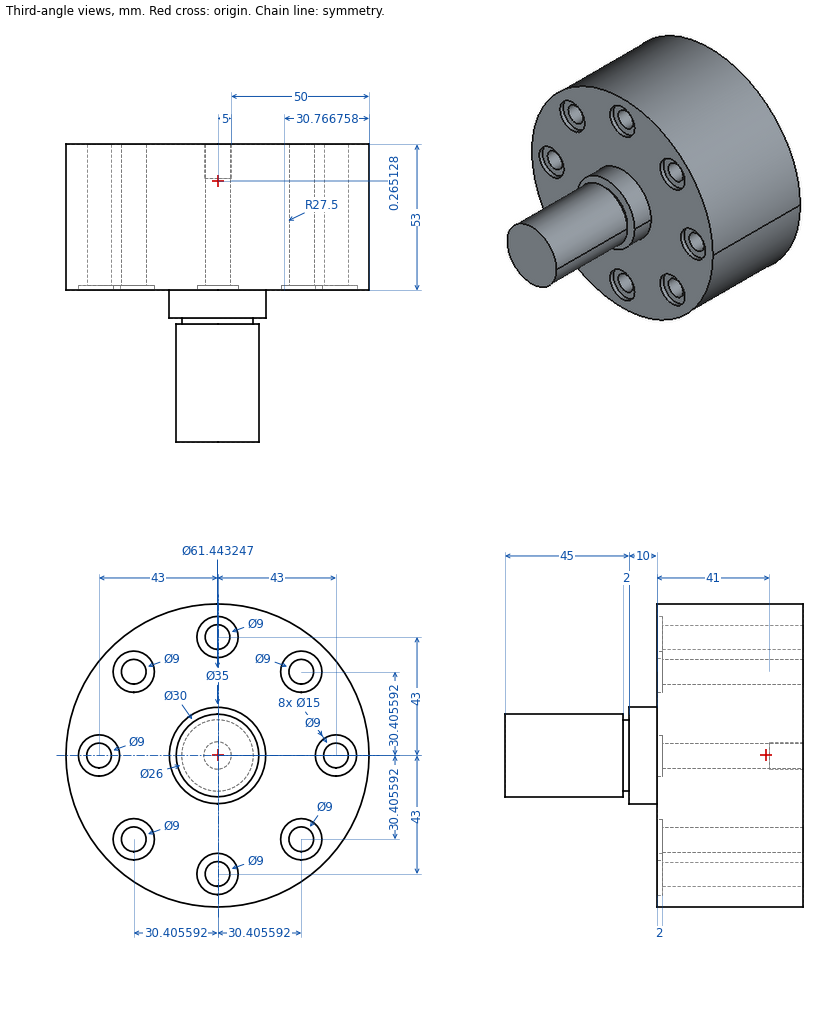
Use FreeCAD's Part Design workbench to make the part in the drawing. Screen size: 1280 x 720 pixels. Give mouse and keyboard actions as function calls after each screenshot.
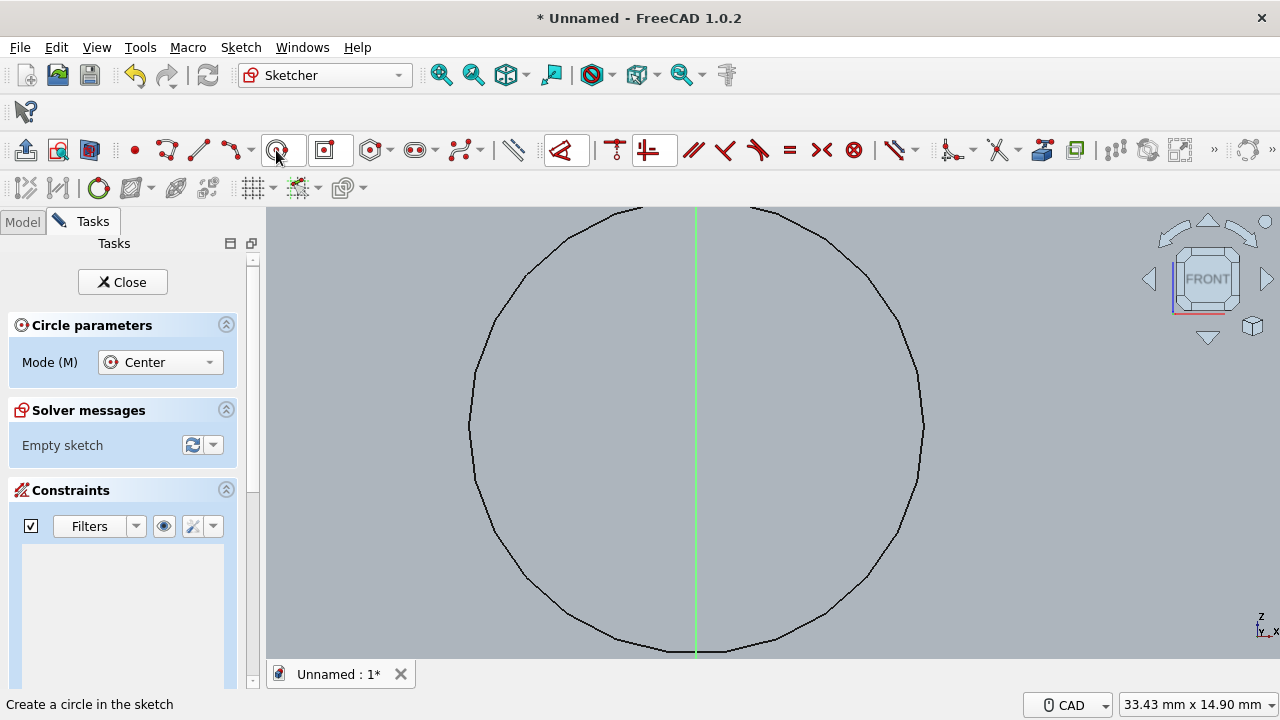
click(696, 426)
move(793, 330)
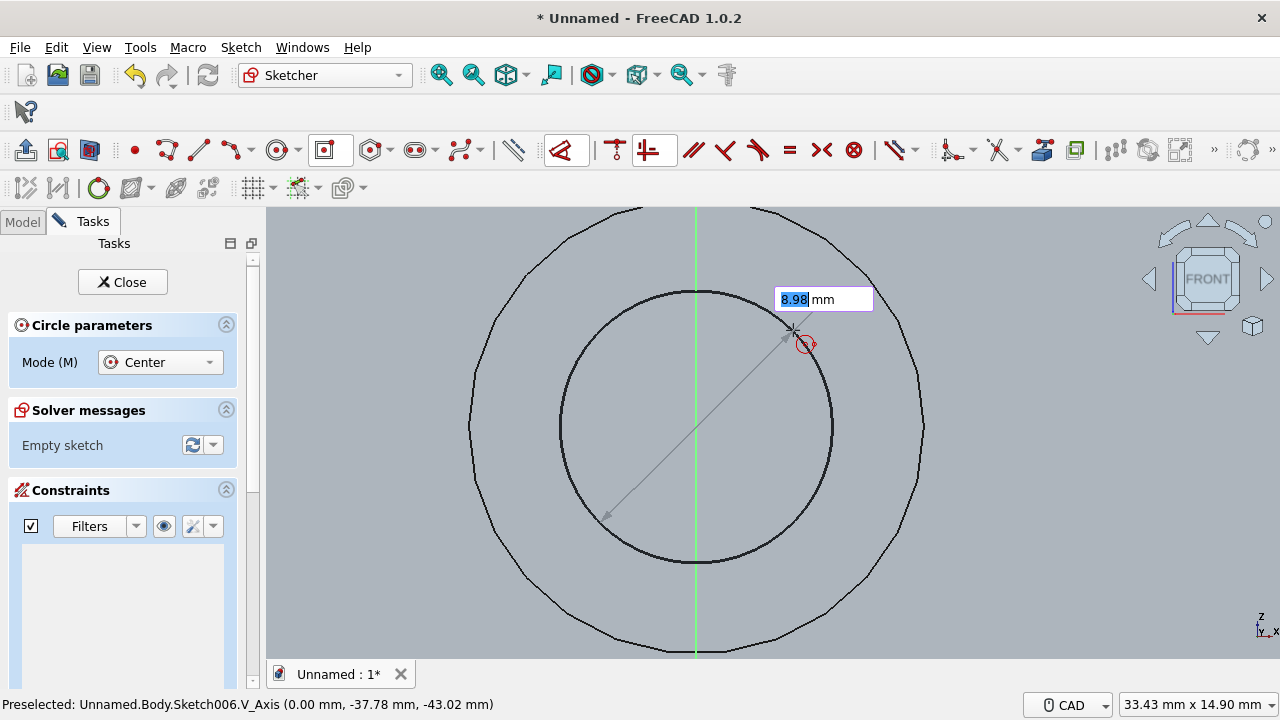
text(9)
key(Return)
key(Escape)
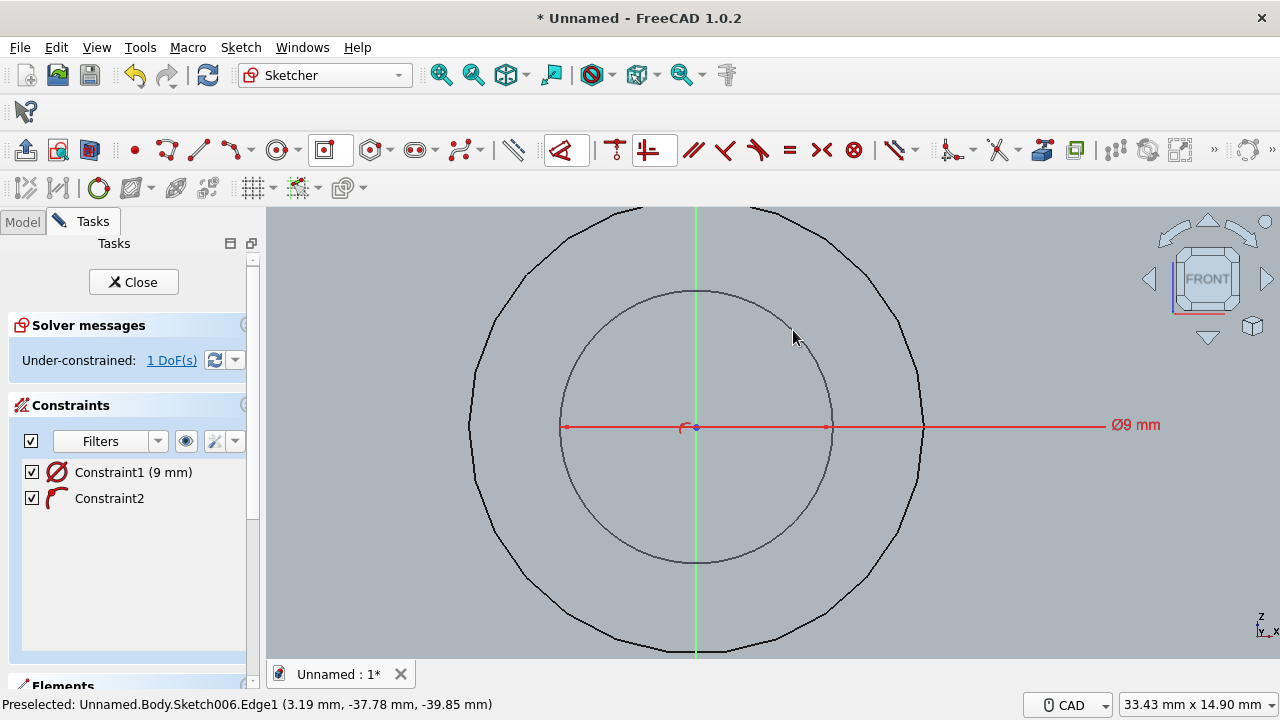
click(696, 427)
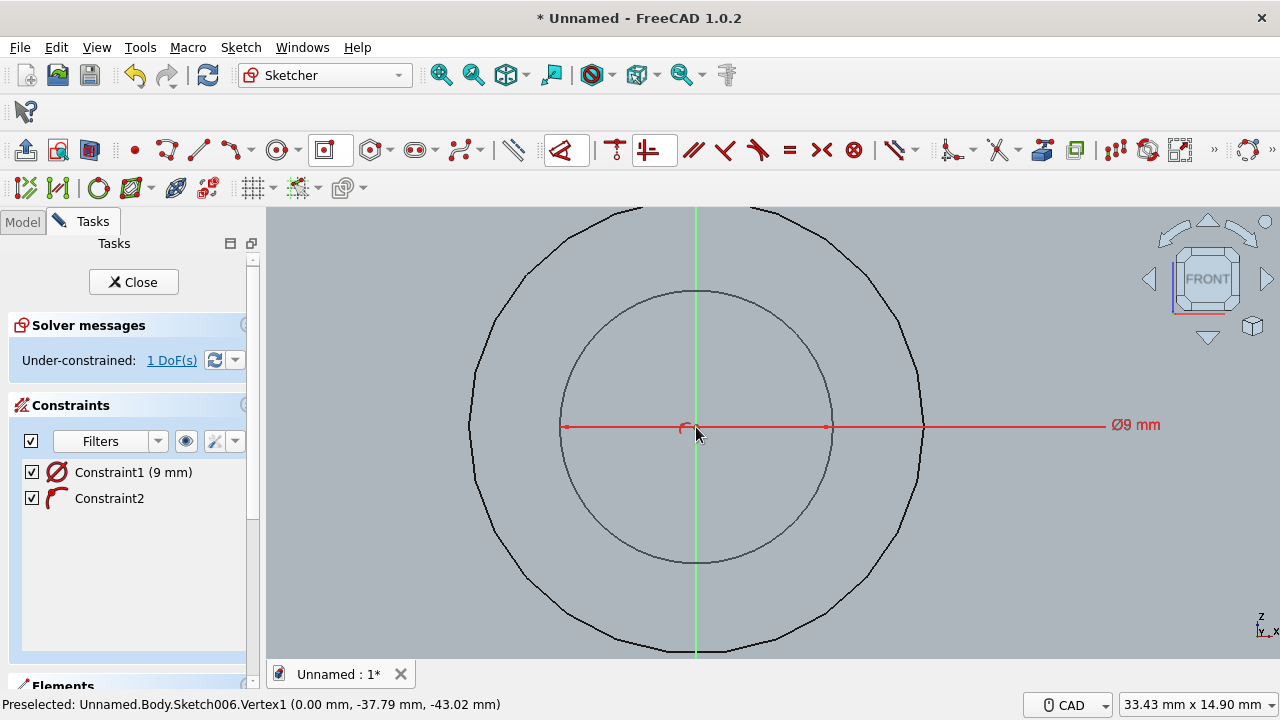
click(584, 150)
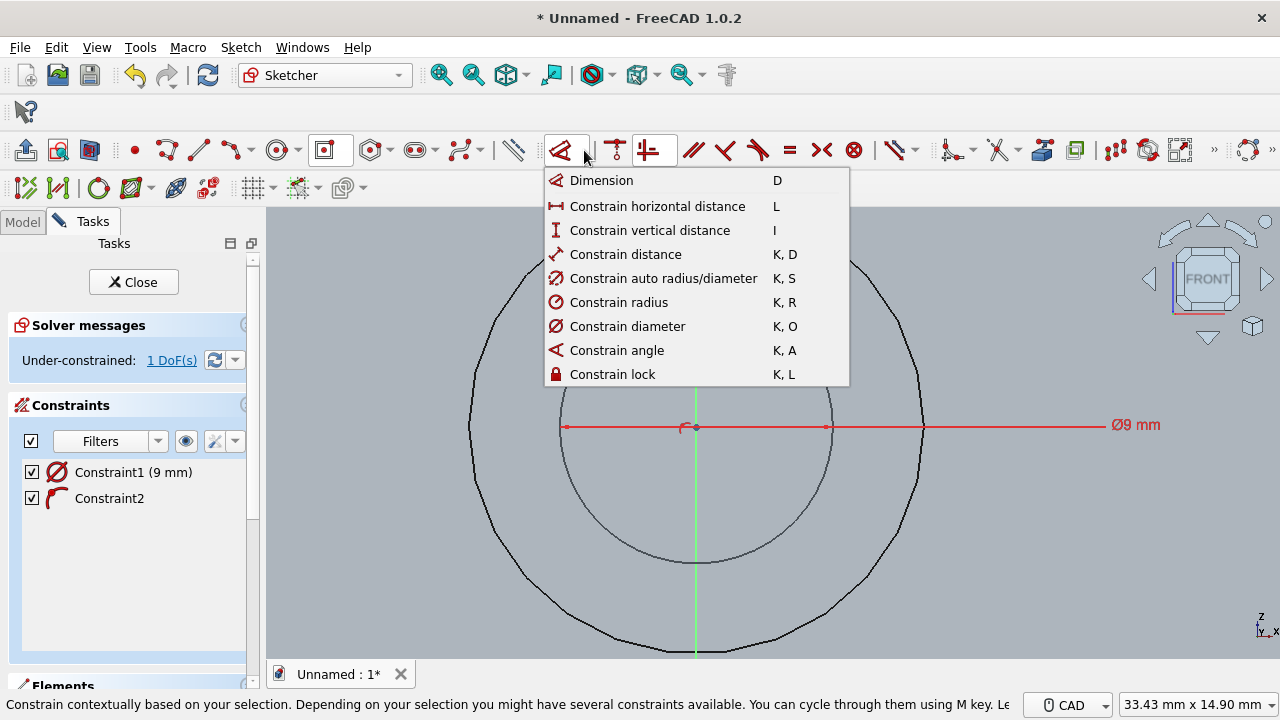
click(697, 230)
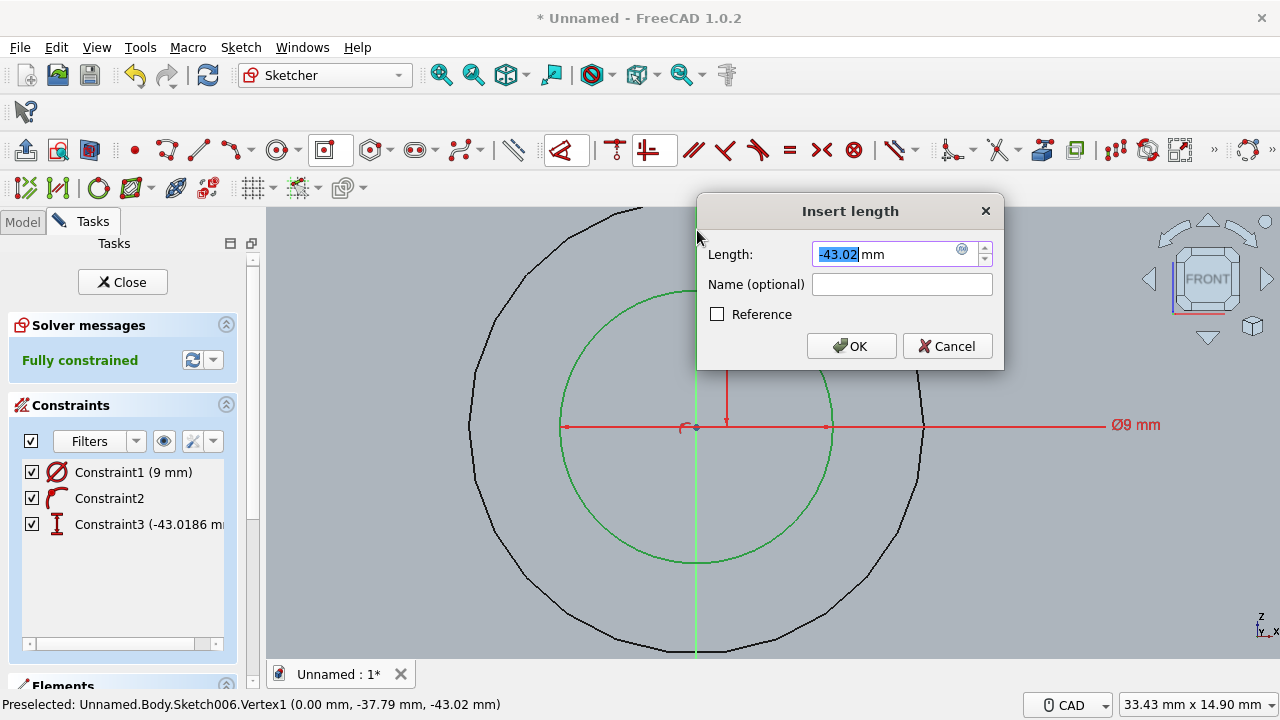
text(-43)
key(Return)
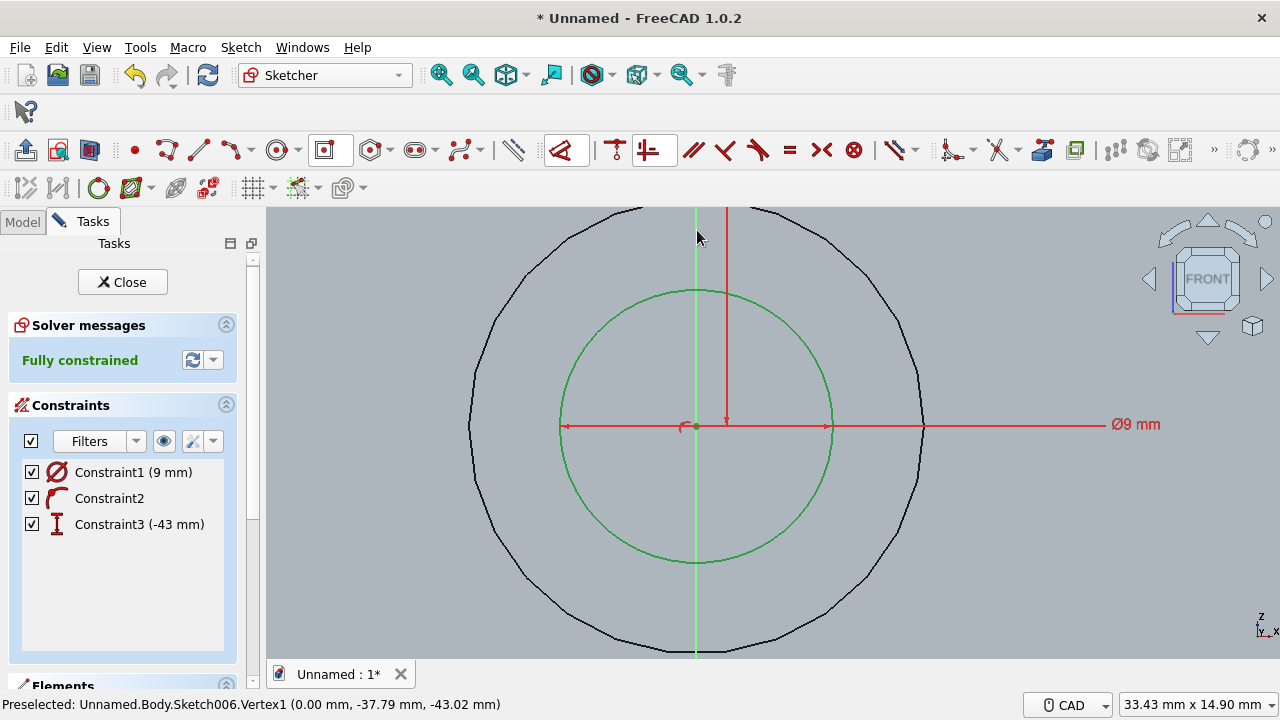
click(123, 282)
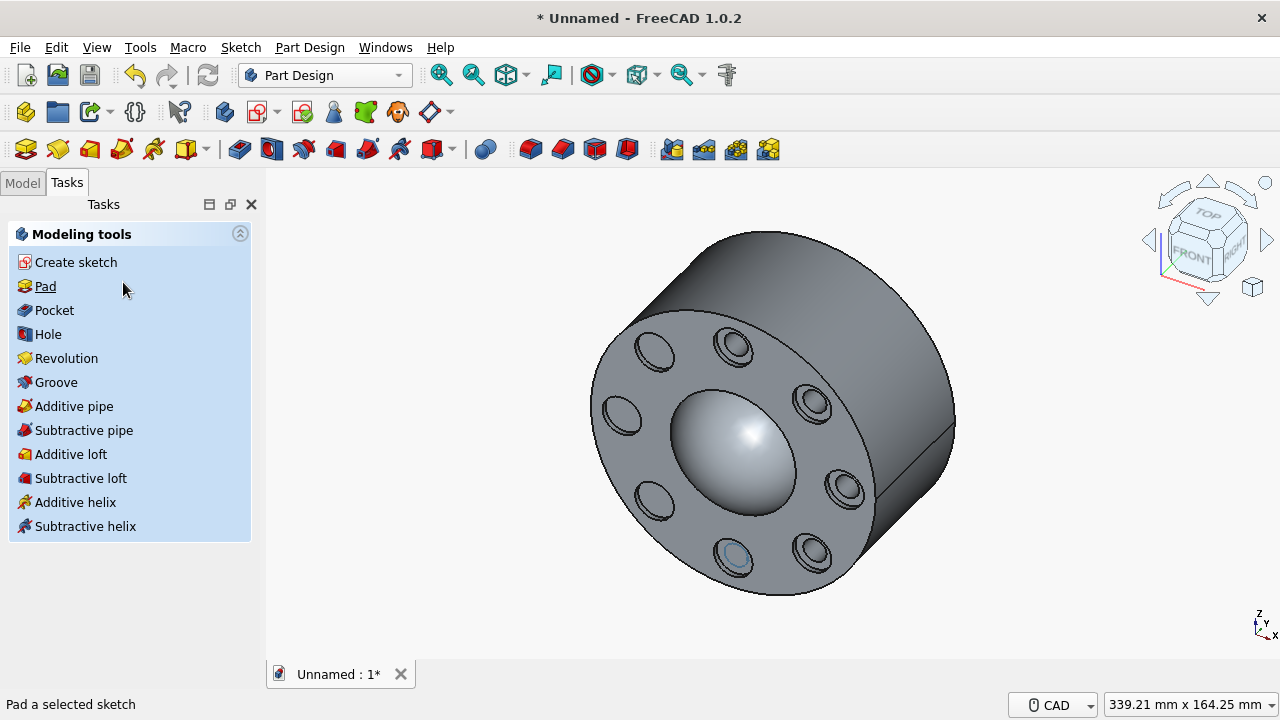
click(240, 150)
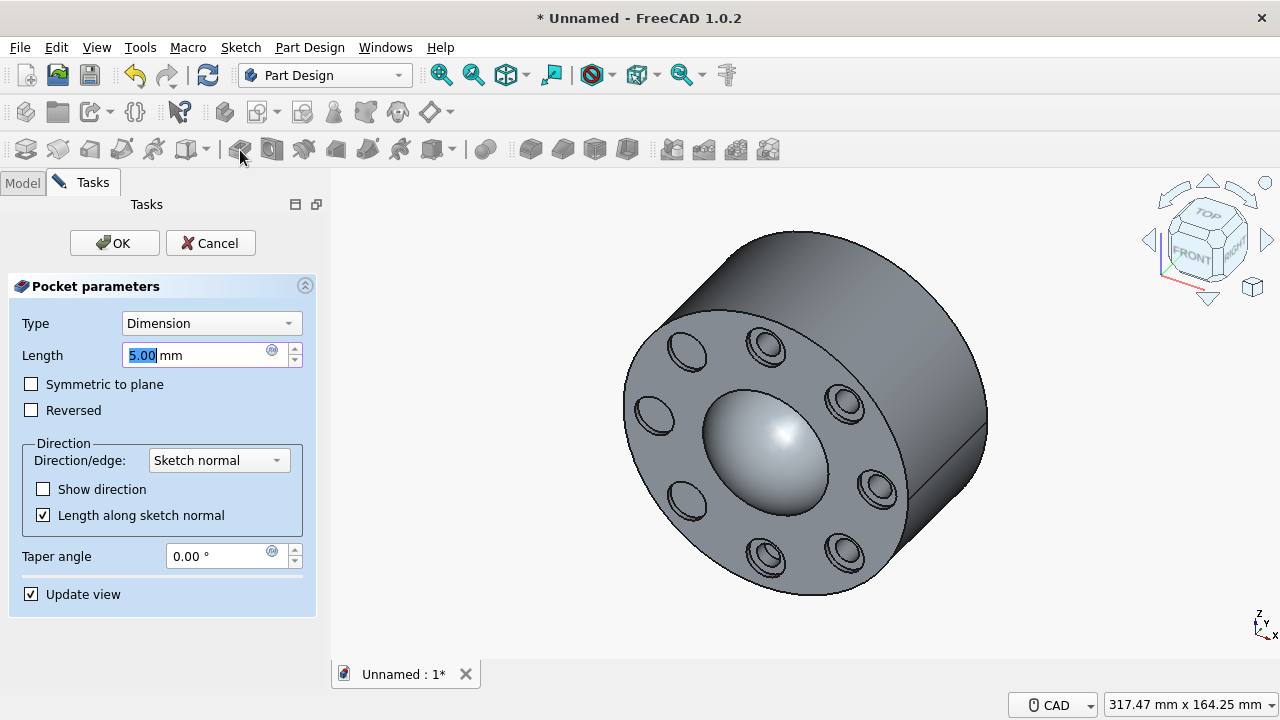
click(212, 324)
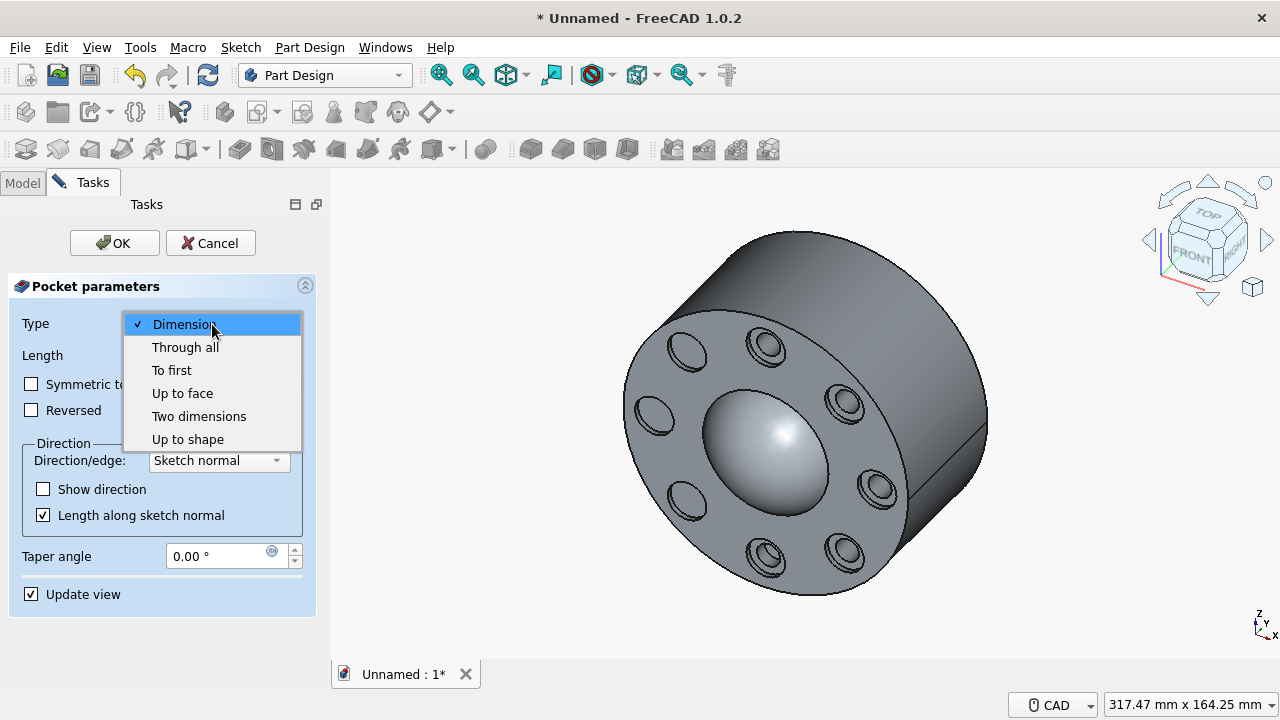
click(212, 370)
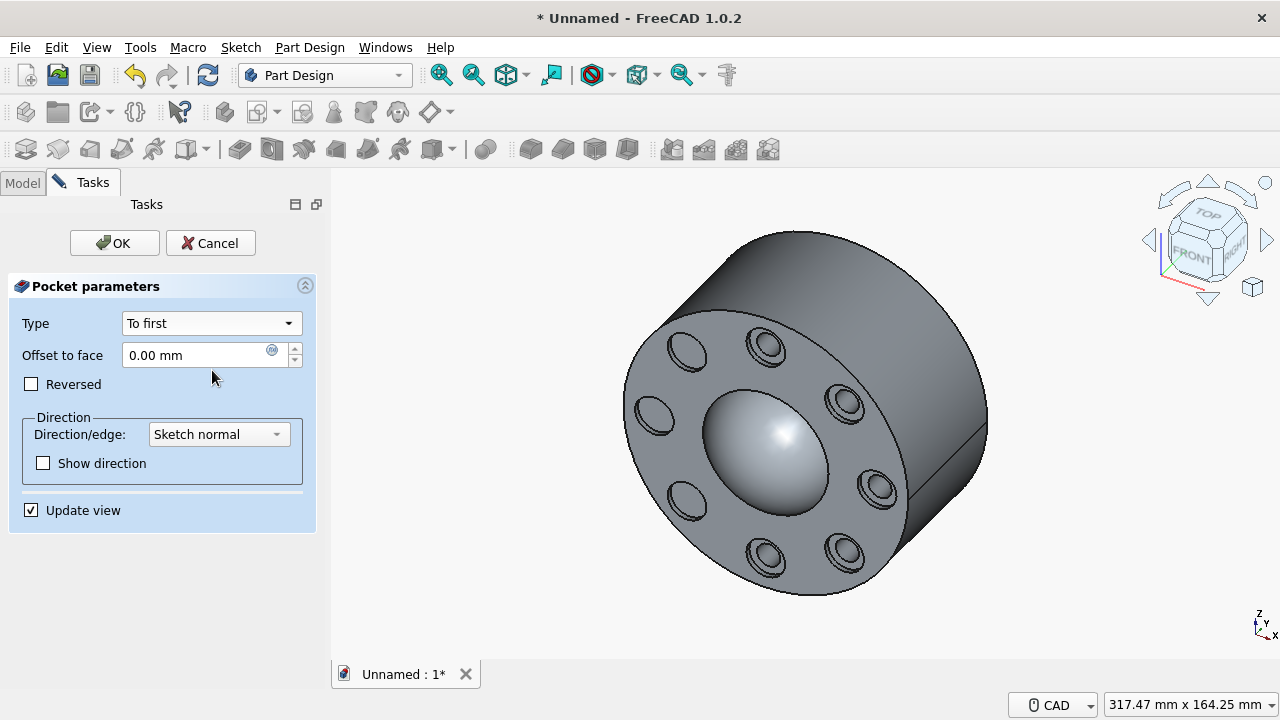
click(115, 243)